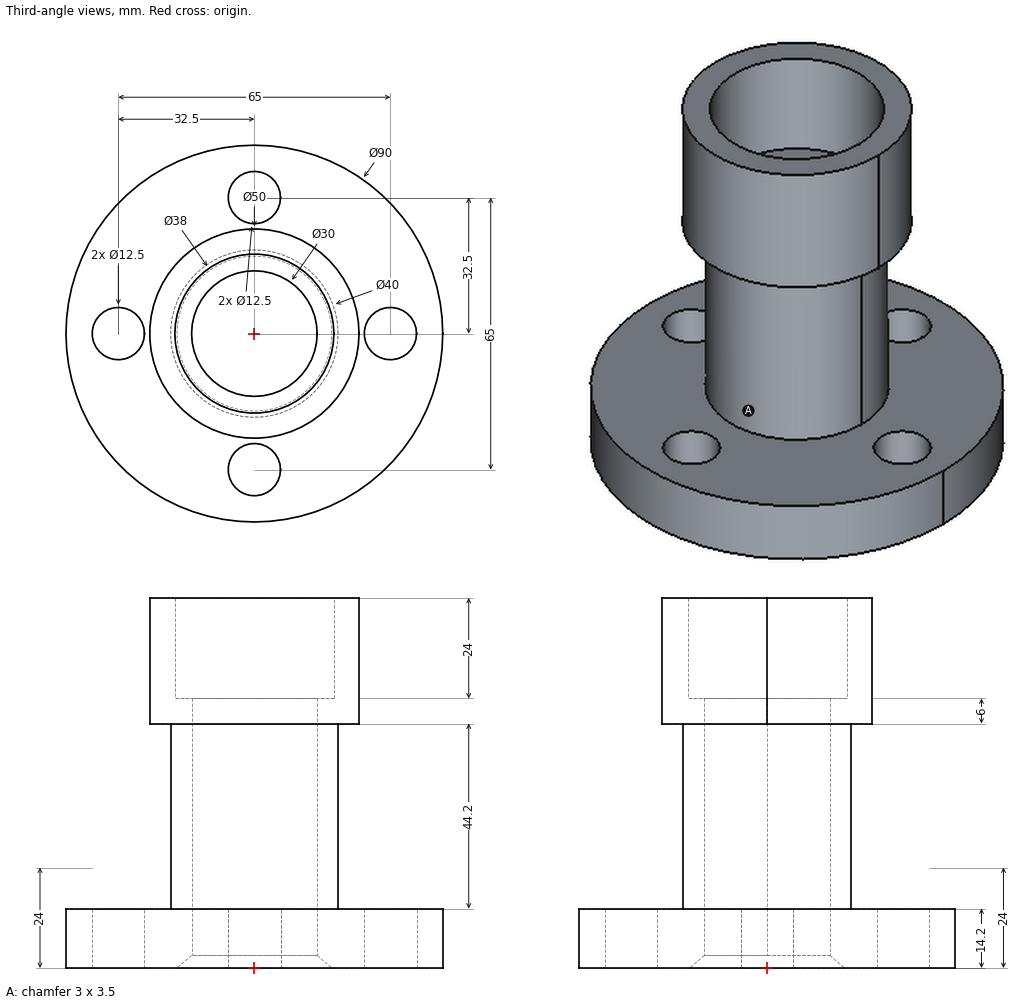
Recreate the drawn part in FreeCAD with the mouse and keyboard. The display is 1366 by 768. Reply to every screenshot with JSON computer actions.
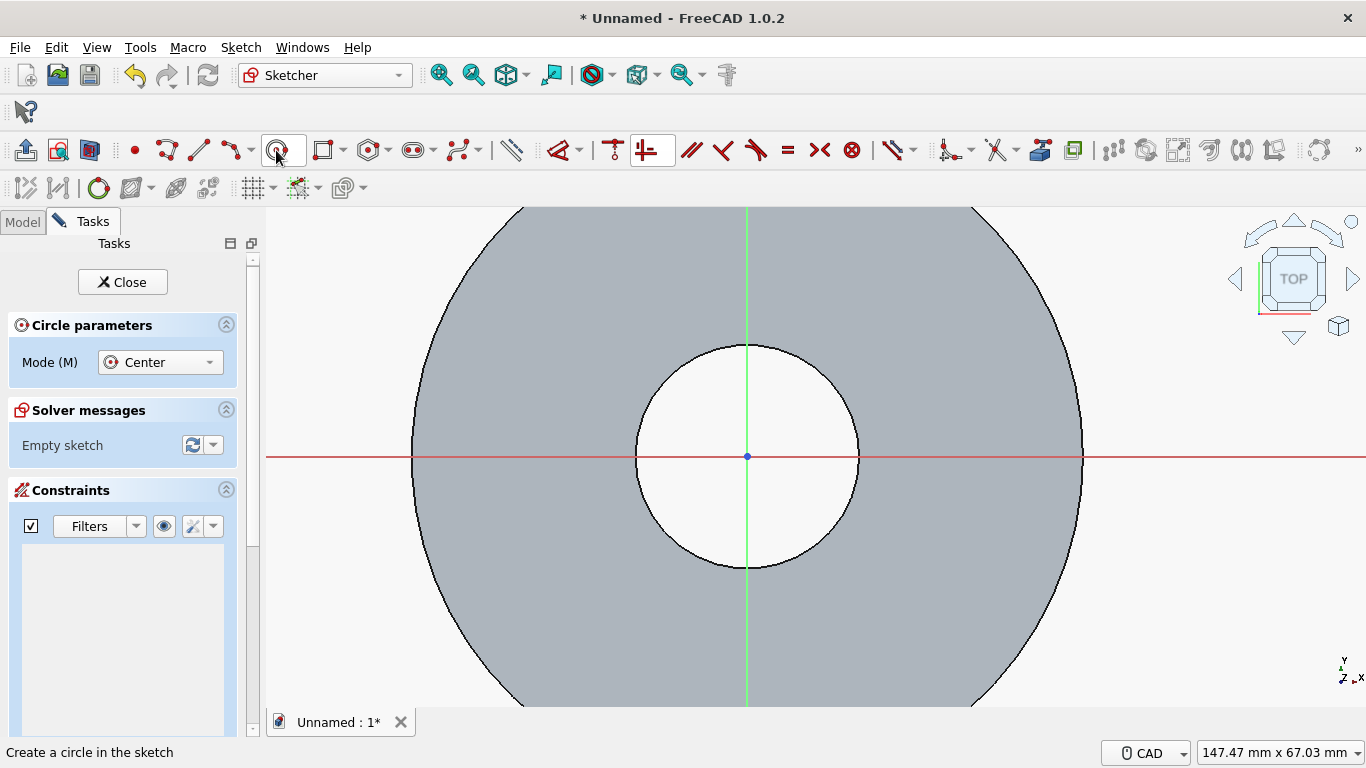
{"action": "left_click", "coordinate": [747, 457]}
{"action": "mouse_move", "coordinate": [853, 351]}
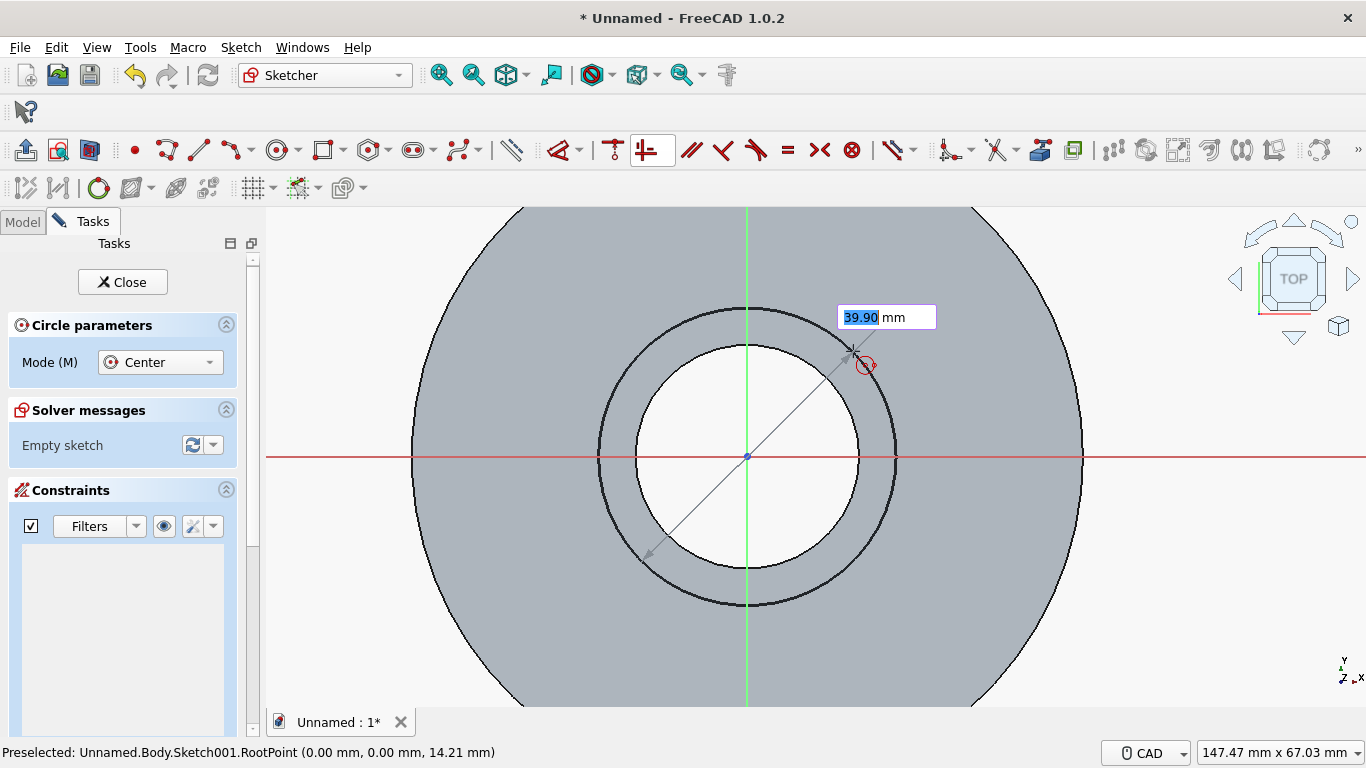
{"action": "type", "text": "40"}
{"action": "key", "text": "Return"}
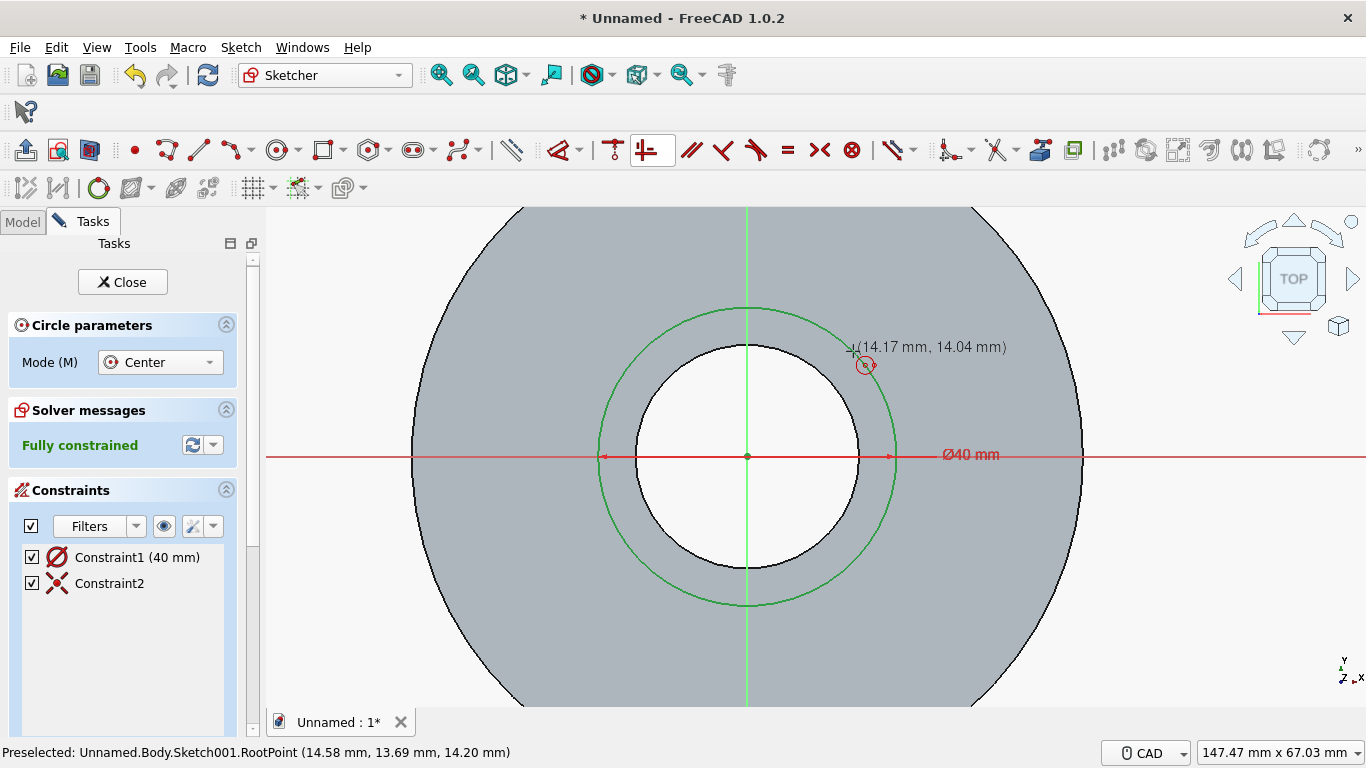
{"action": "left_click", "coordinate": [747, 457]}
{"action": "mouse_move", "coordinate": [826, 378]}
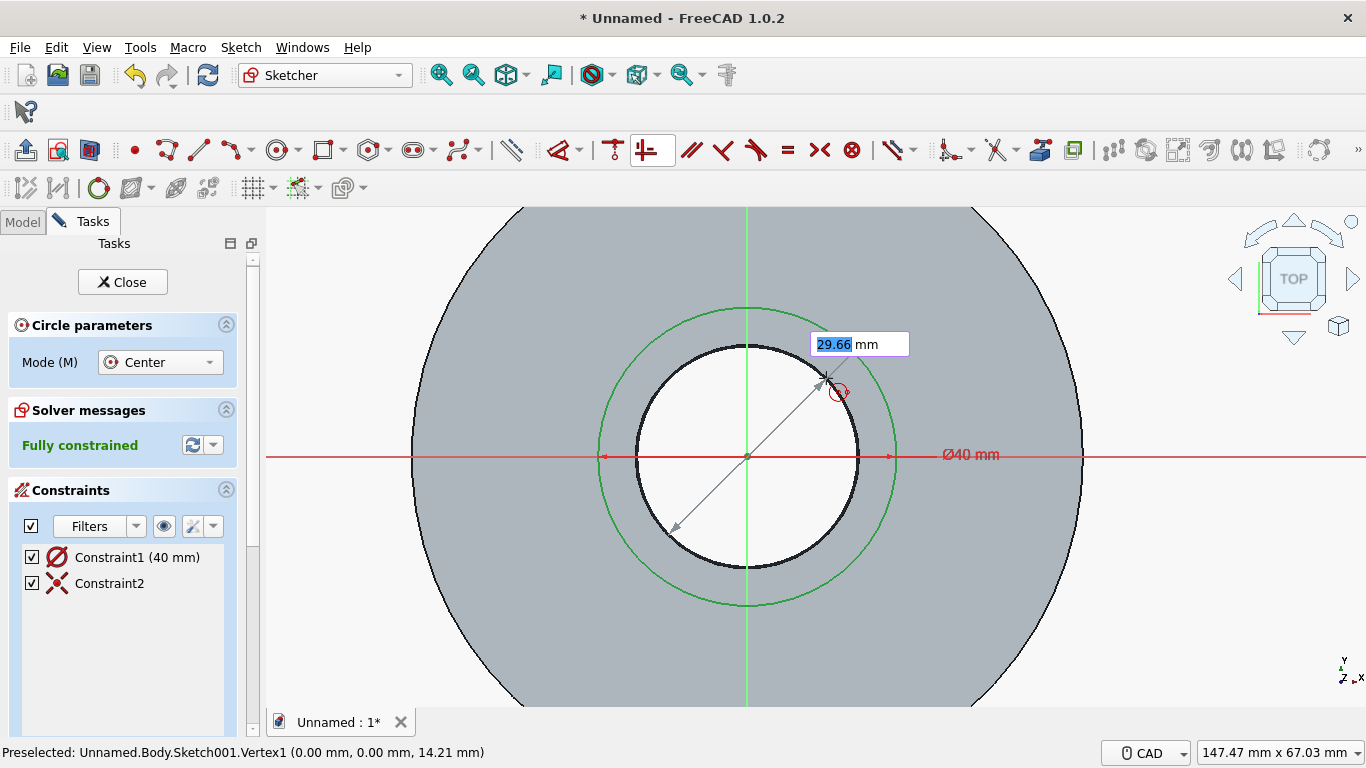
{"action": "type", "text": "30"}
{"action": "key", "text": "Return"}
{"action": "key", "text": "Escape"}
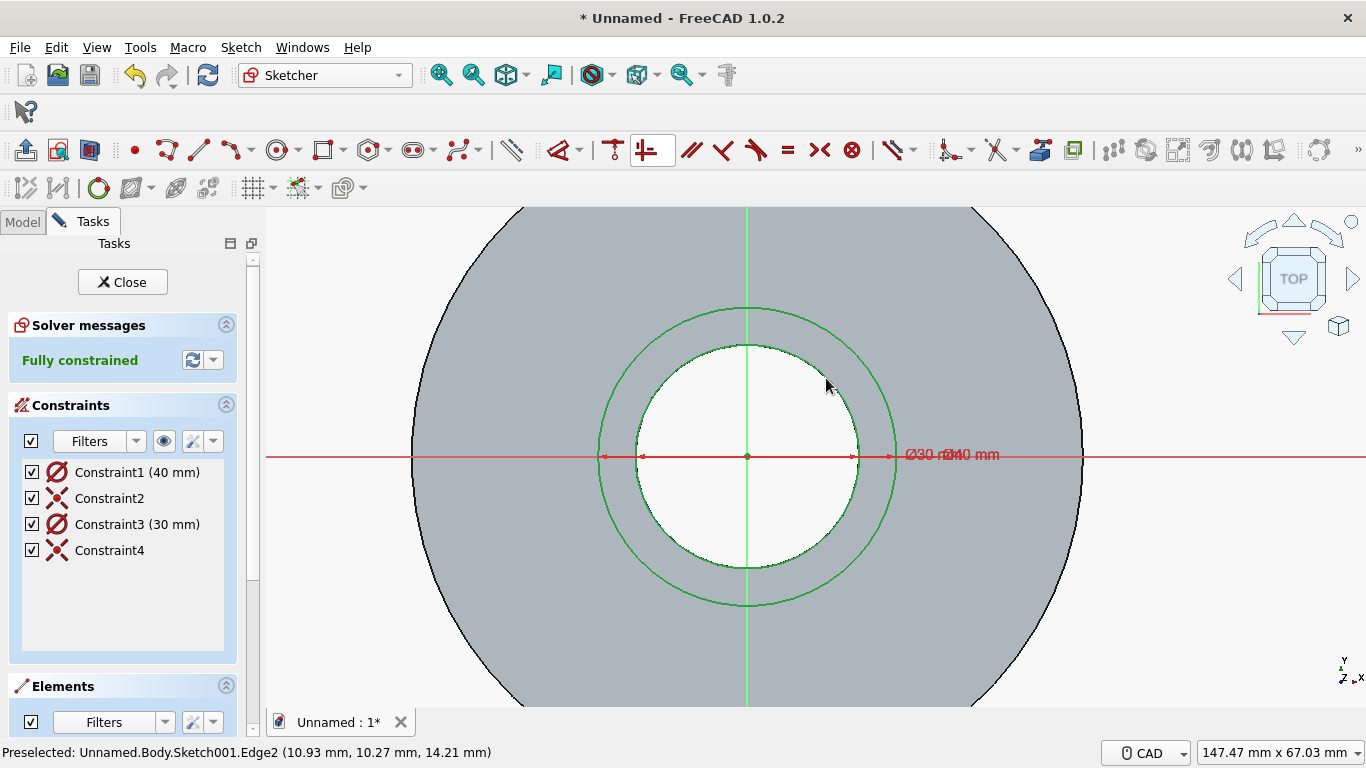
{"action": "left_click", "coordinate": [123, 282]}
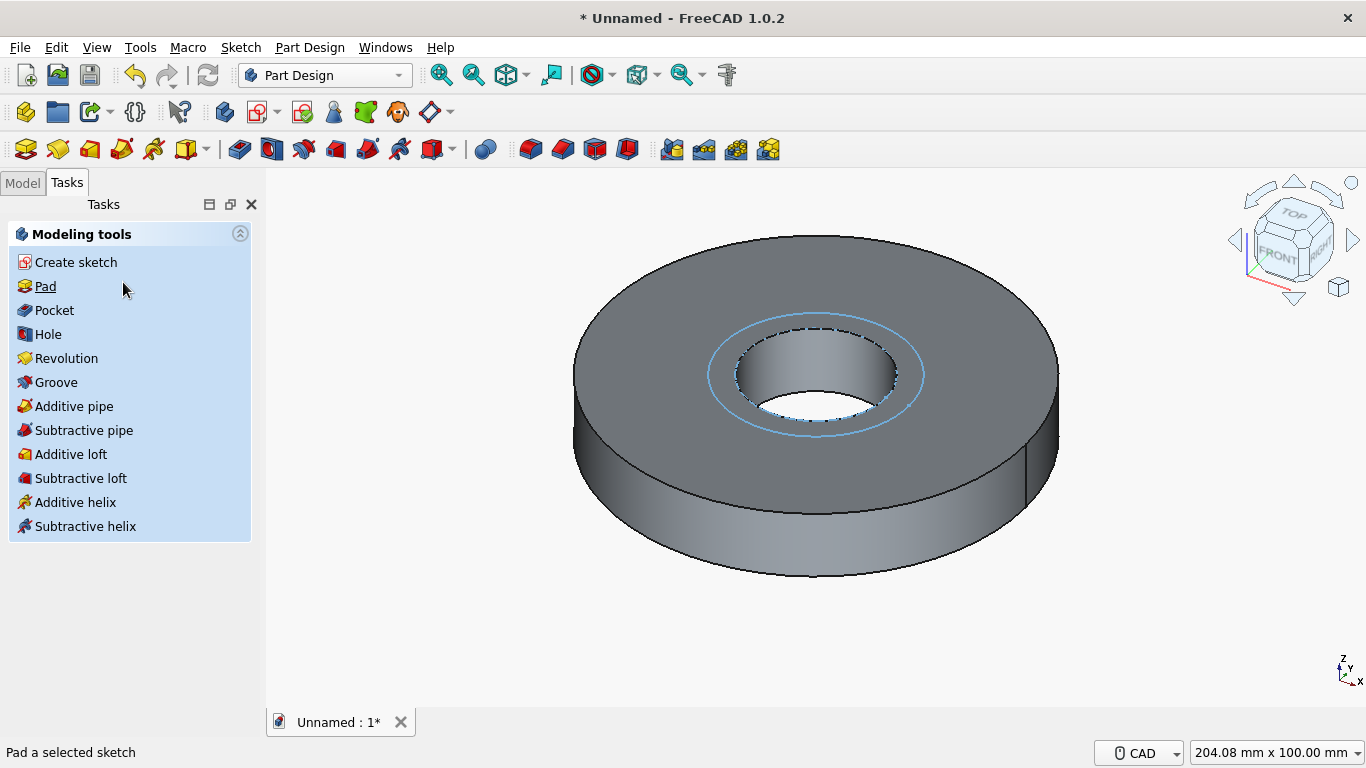
{"action": "left_click", "coordinate": [26, 150]}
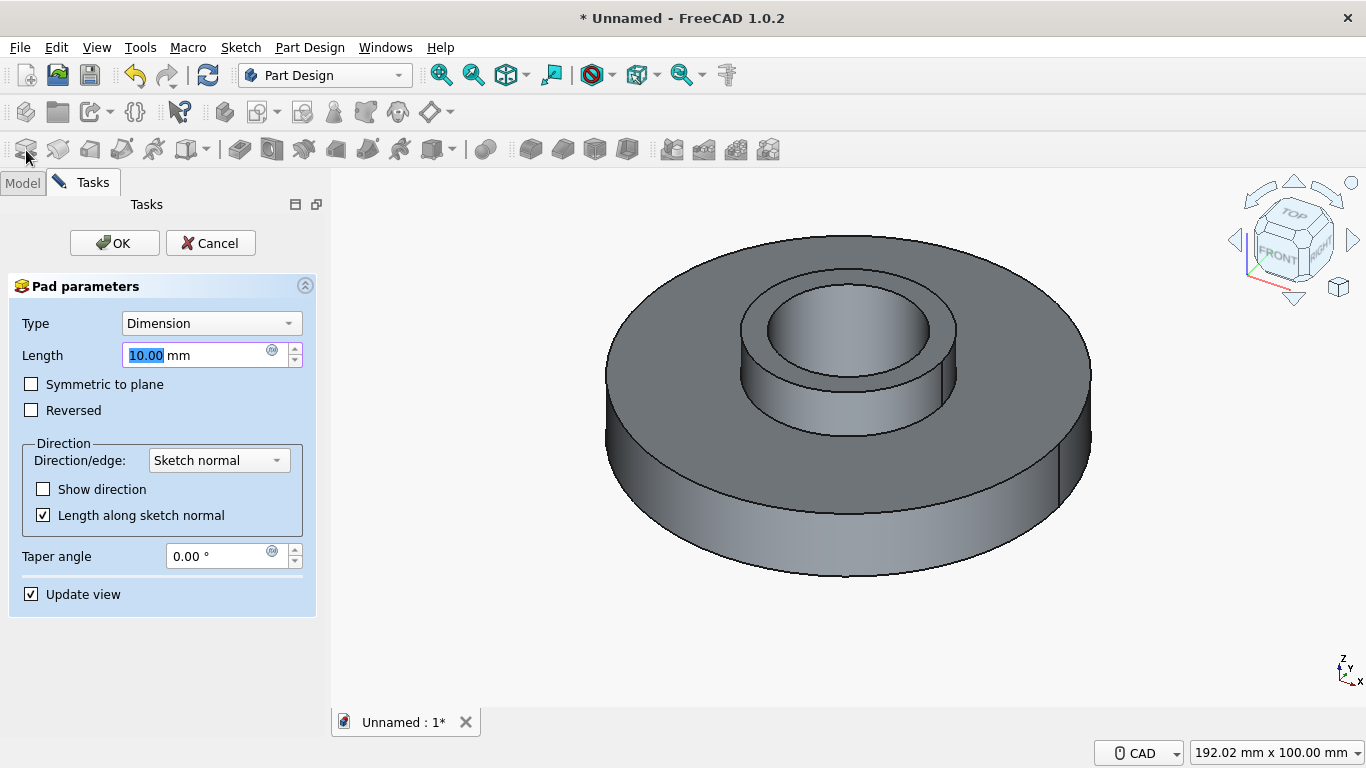
{"action": "type", "text": "44.2"}
{"action": "key", "text": "Tab"}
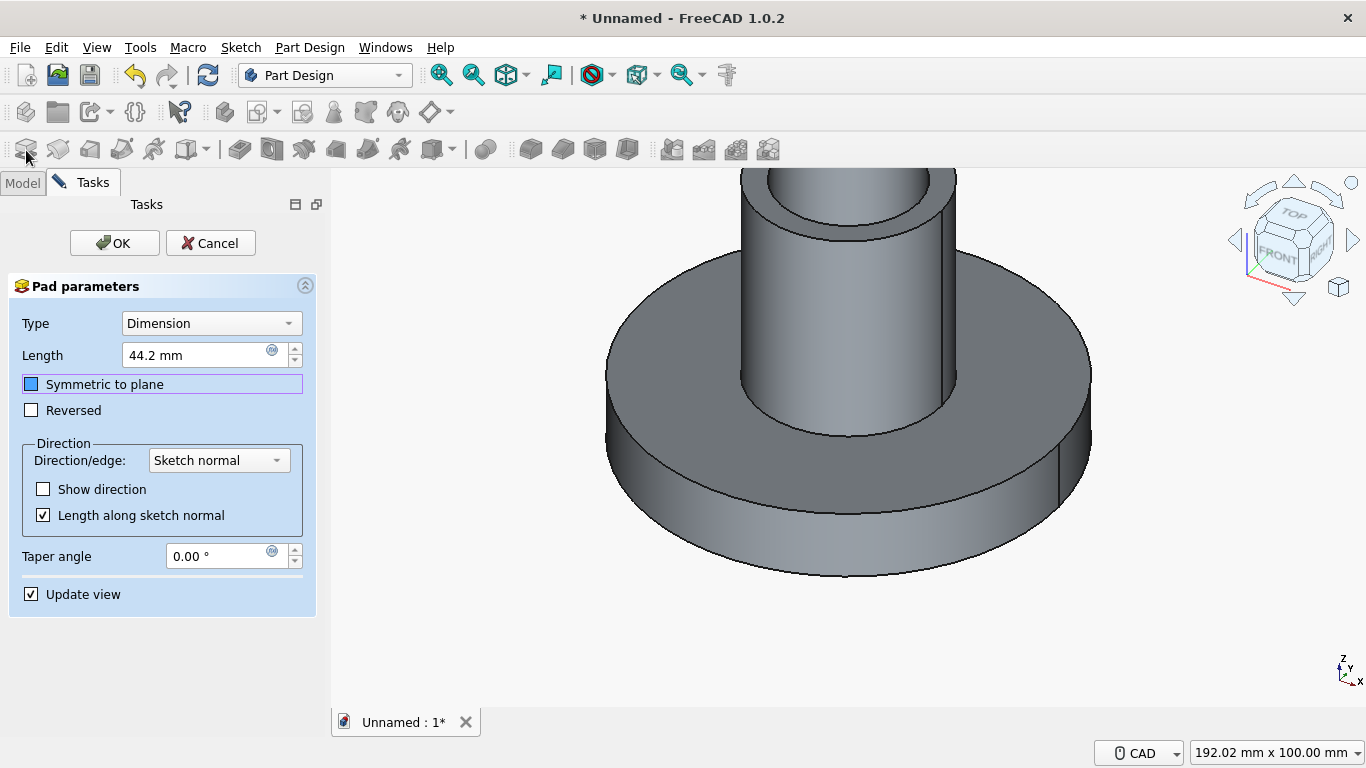
{"action": "left_click", "coordinate": [115, 243]}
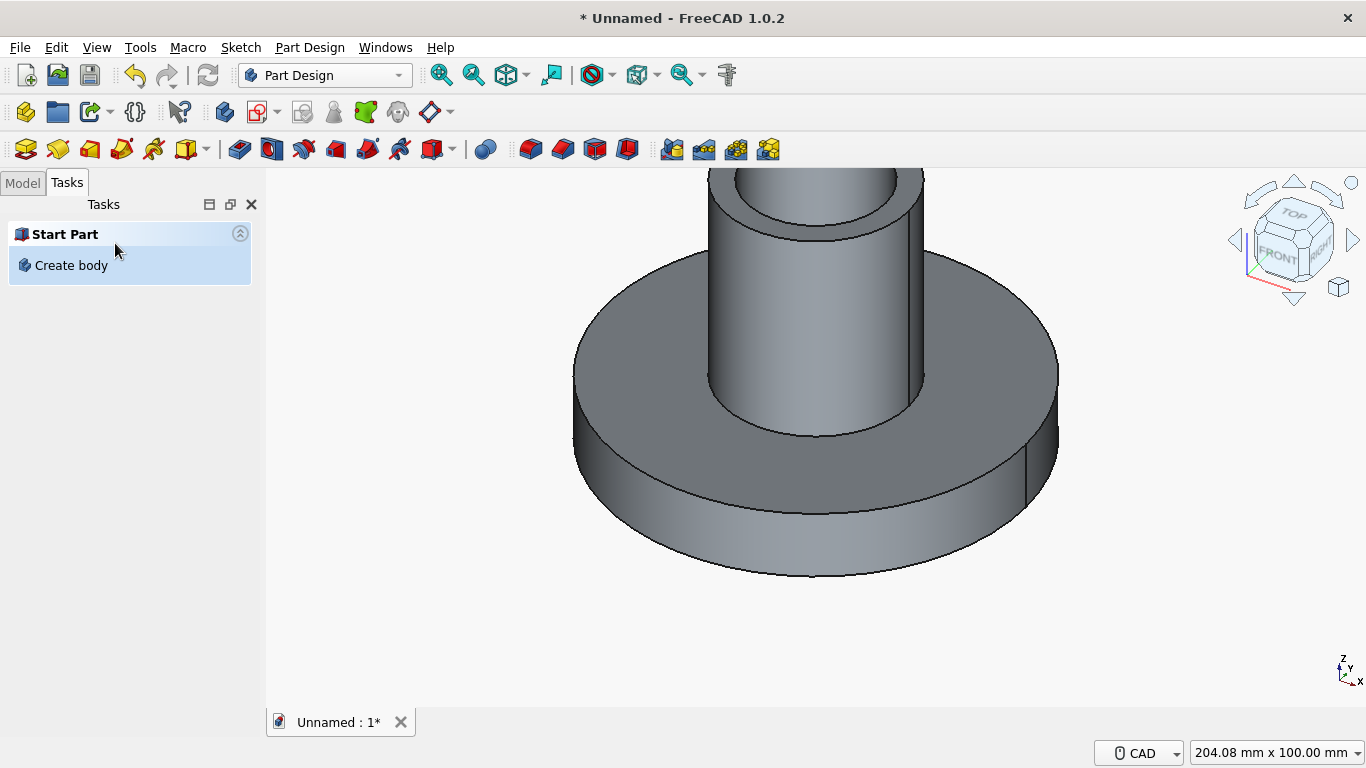
{"action": "key", "text": "v f"}